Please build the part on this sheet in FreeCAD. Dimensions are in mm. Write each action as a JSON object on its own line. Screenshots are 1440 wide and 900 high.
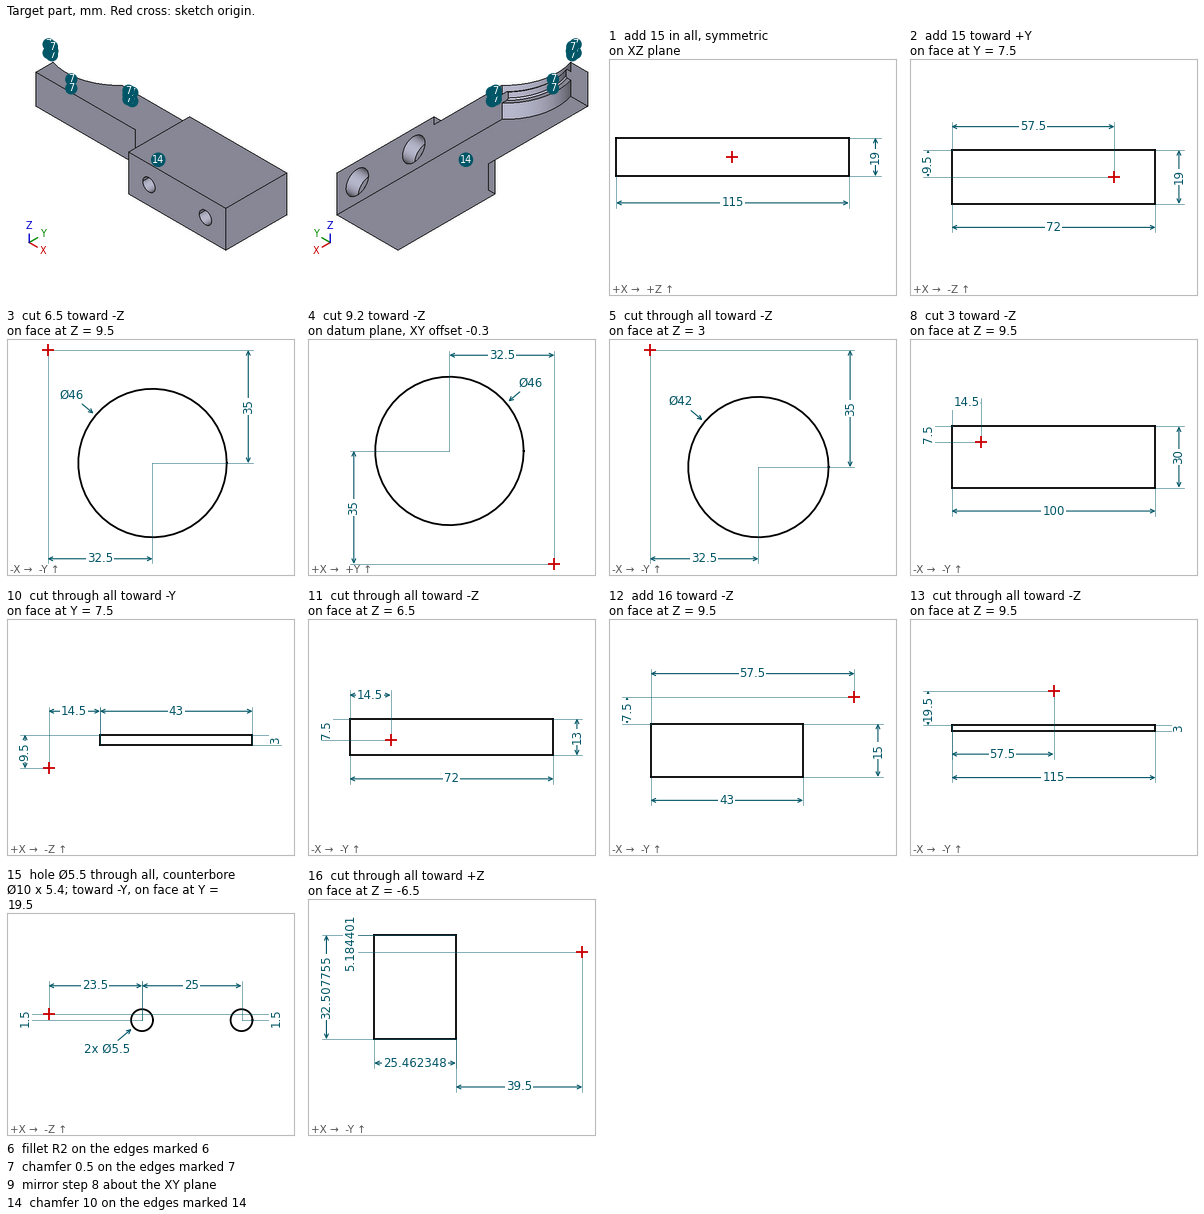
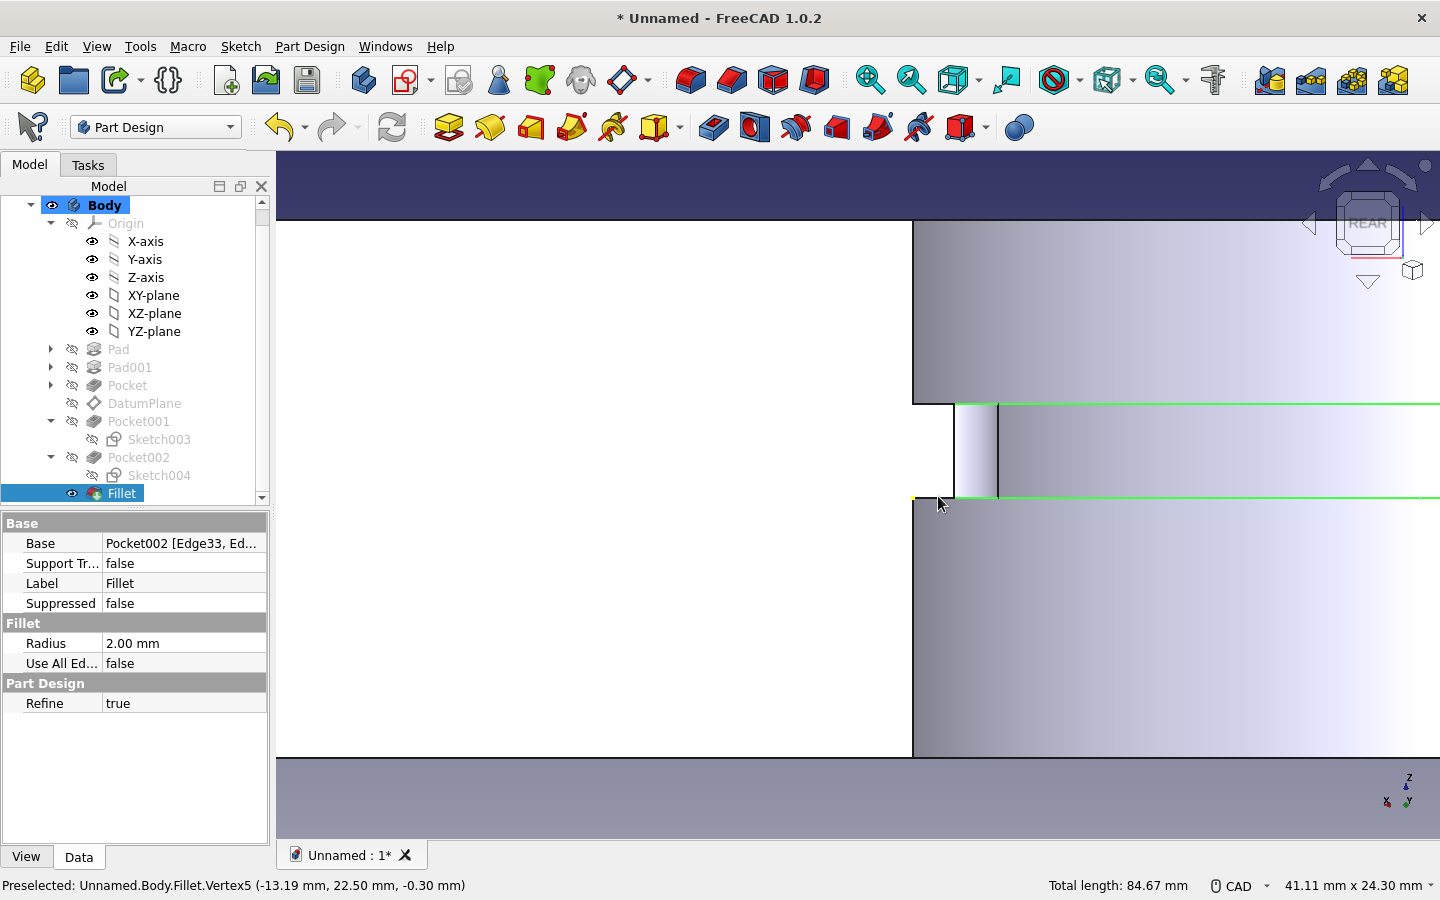
{"action": "left_click", "coordinate": [934, 497], "text": "ctrl"}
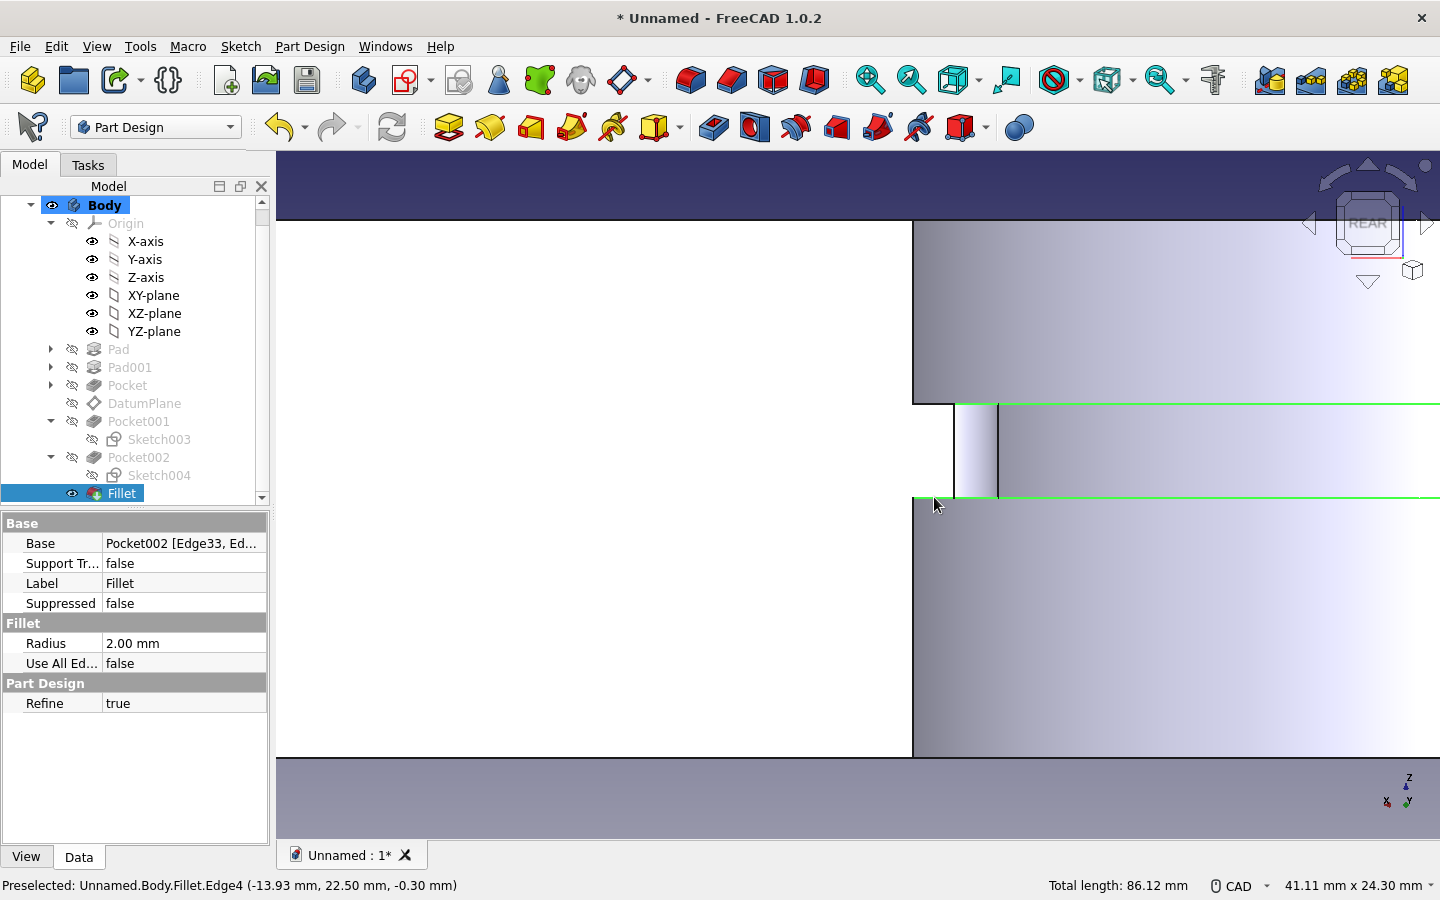
{"action": "left_click", "coordinate": [871, 80]}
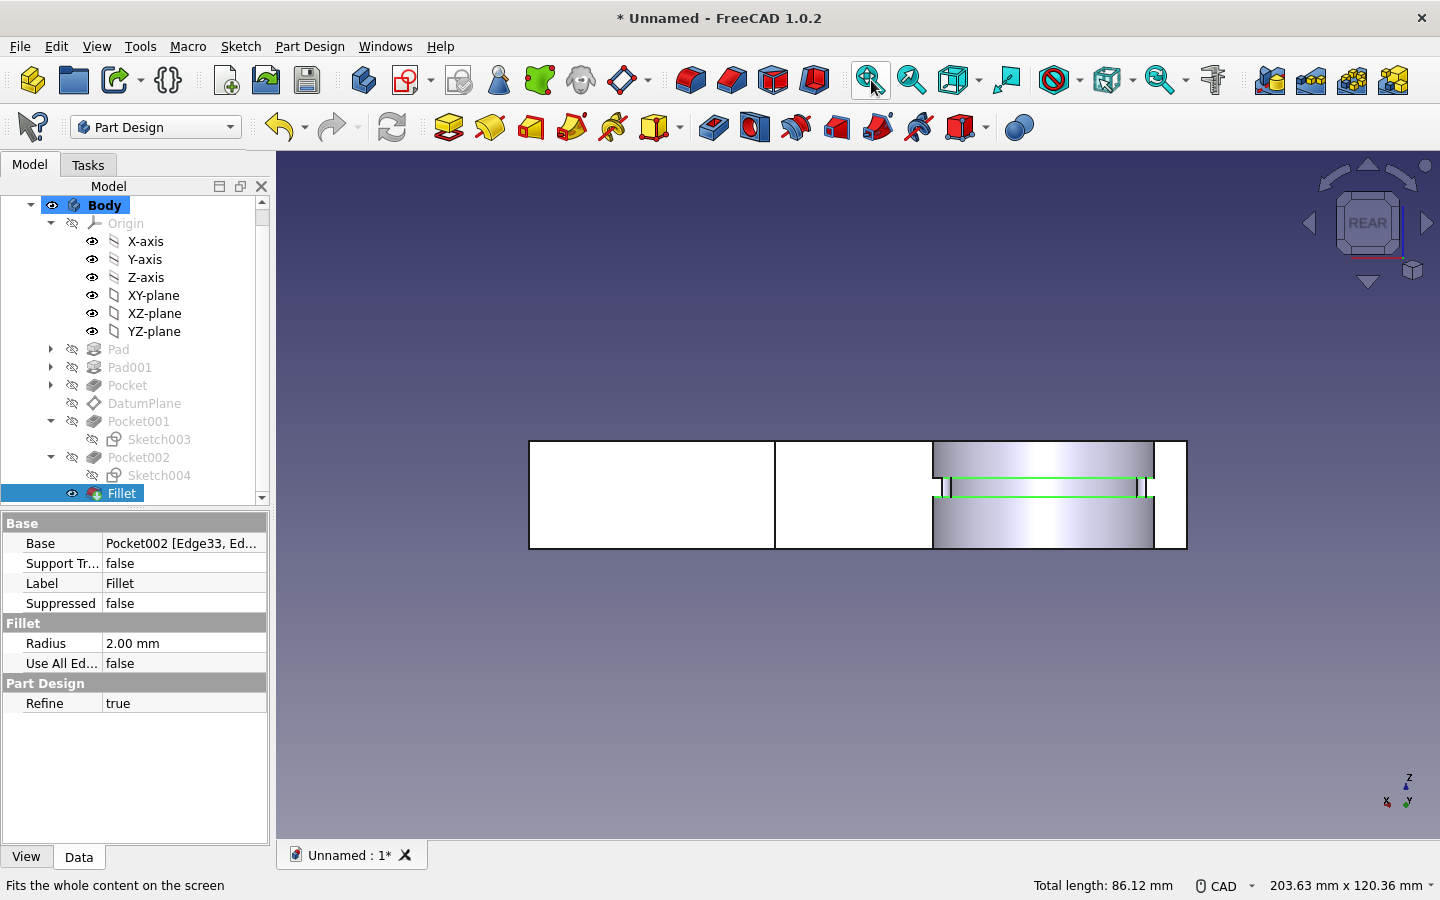
{"action": "key", "text": "6"}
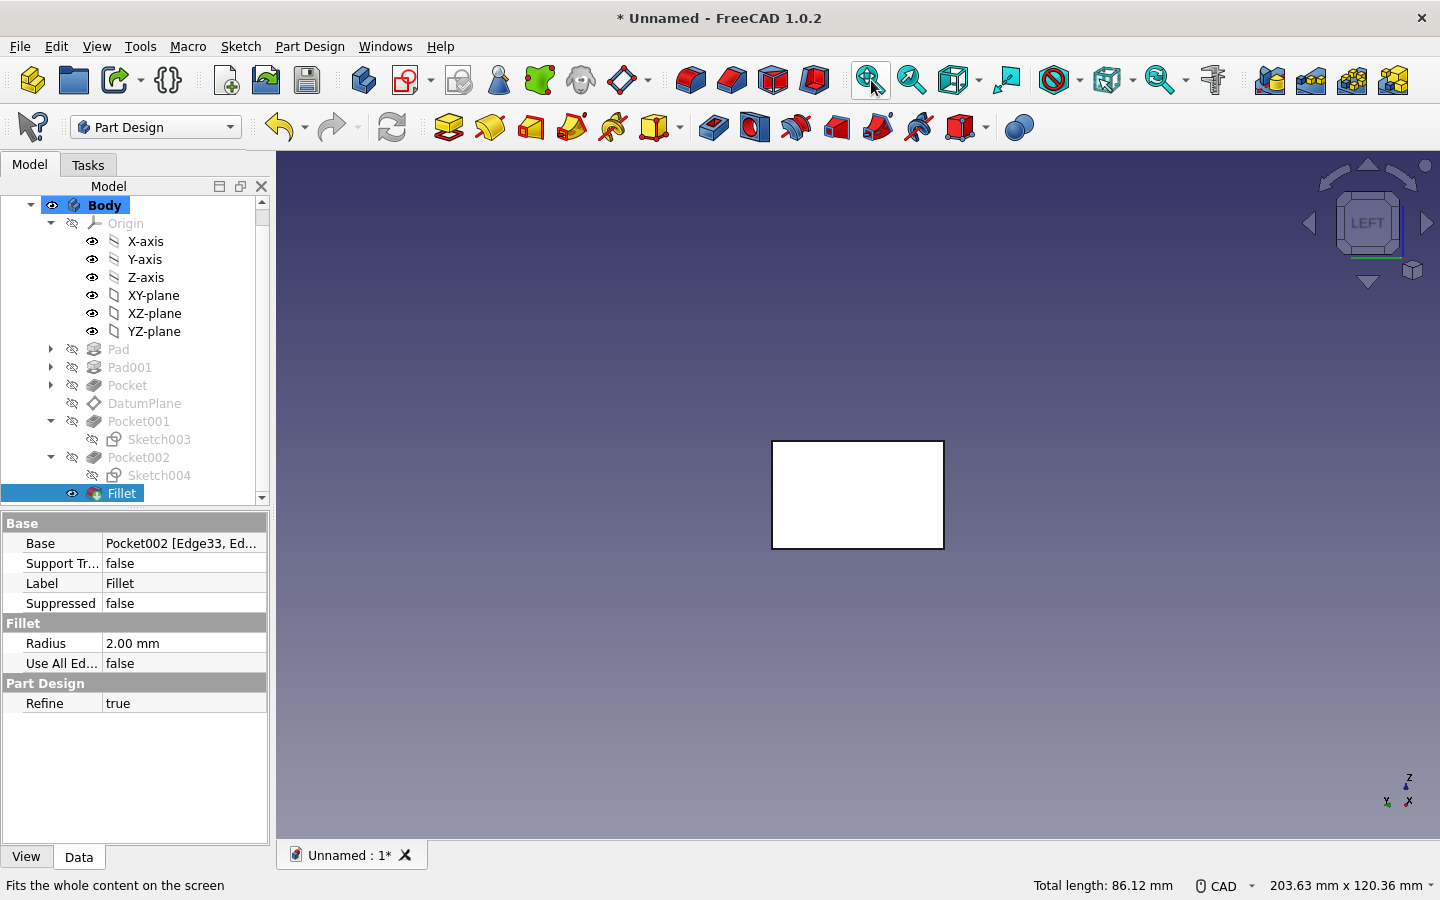
{"action": "left_click", "coordinate": [871, 80]}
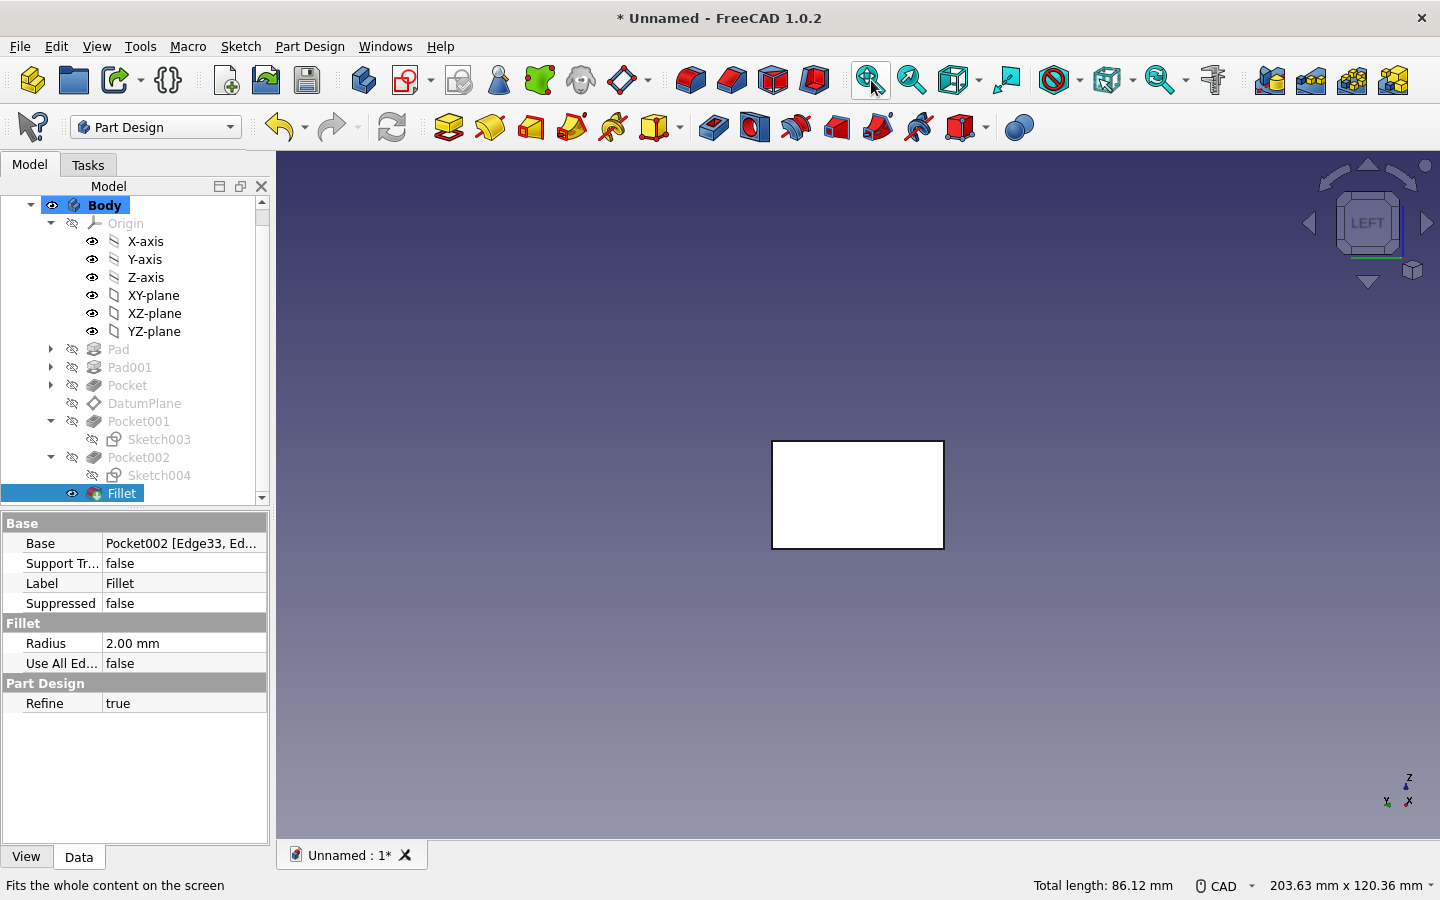
{"action": "scroll", "coordinate": [772, 477], "scroll_direction": "up", "scroll_amount": 8}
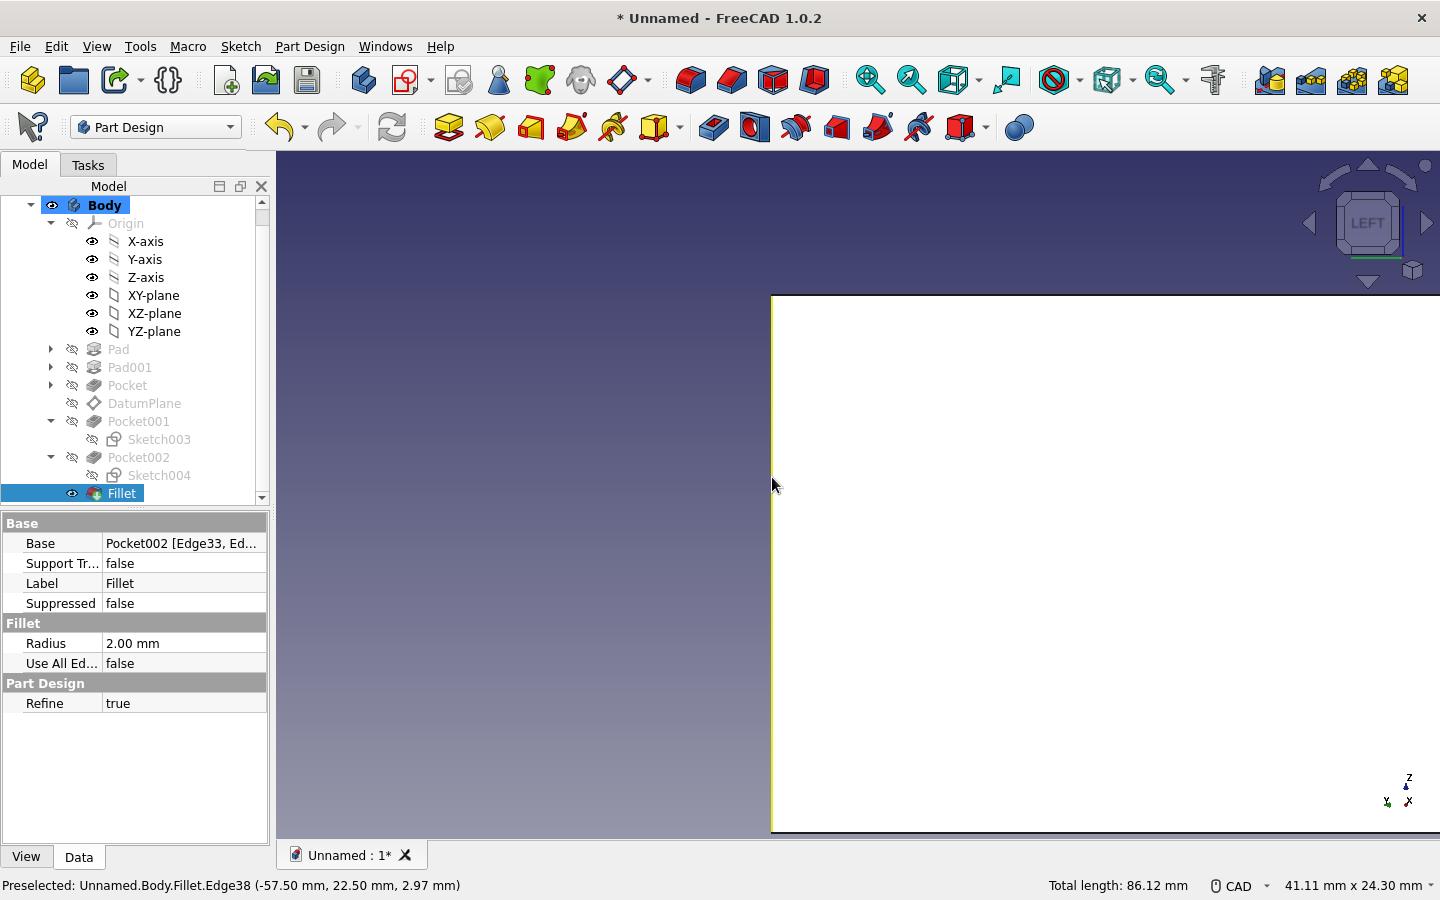
{"action": "left_click", "coordinate": [871, 80]}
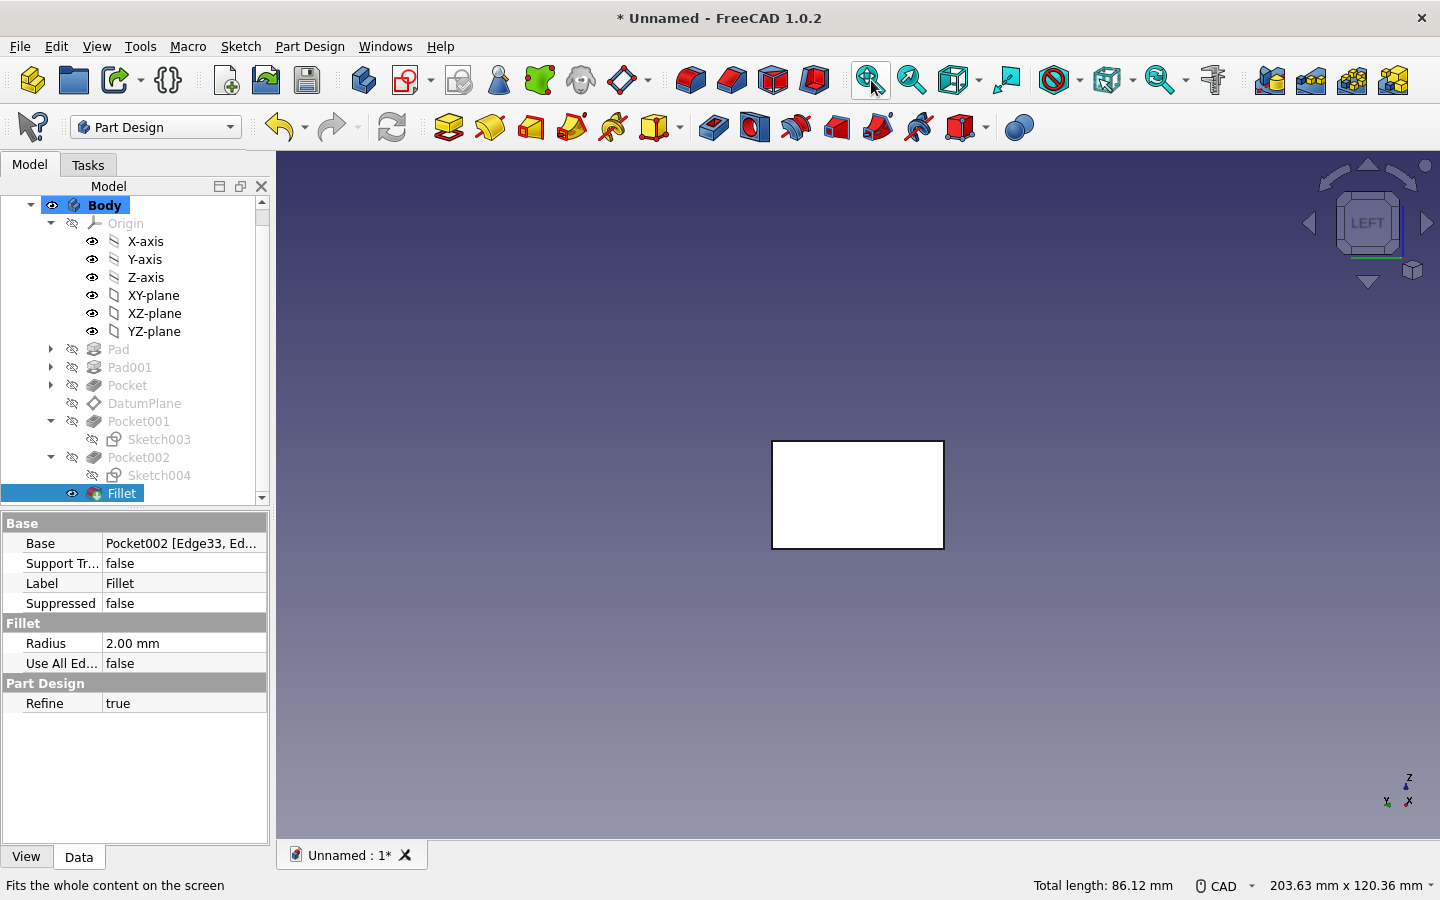
{"action": "key", "text": "v 3"}